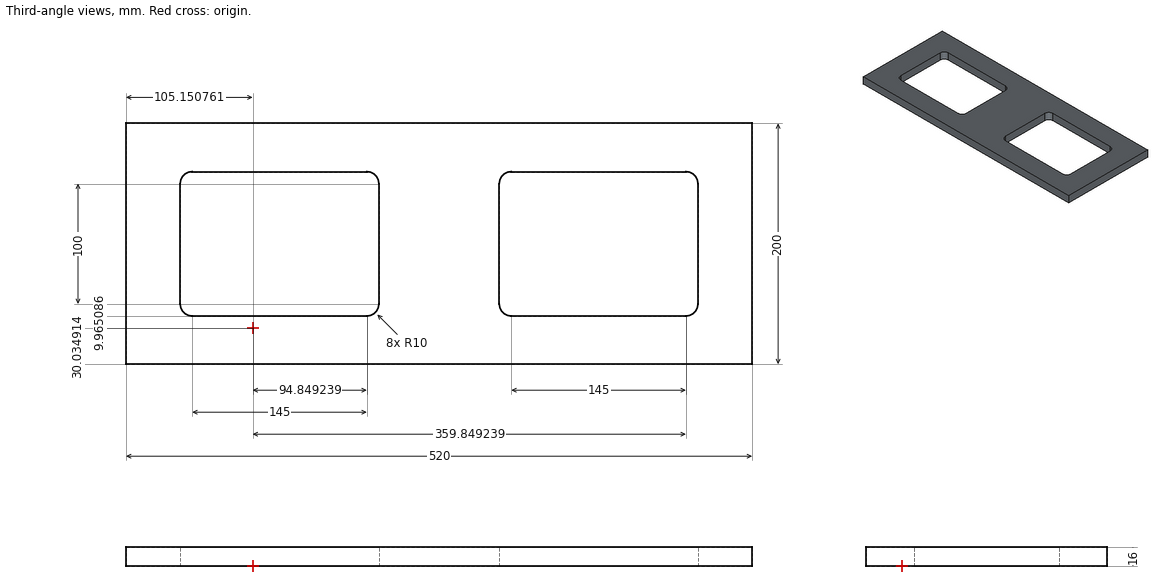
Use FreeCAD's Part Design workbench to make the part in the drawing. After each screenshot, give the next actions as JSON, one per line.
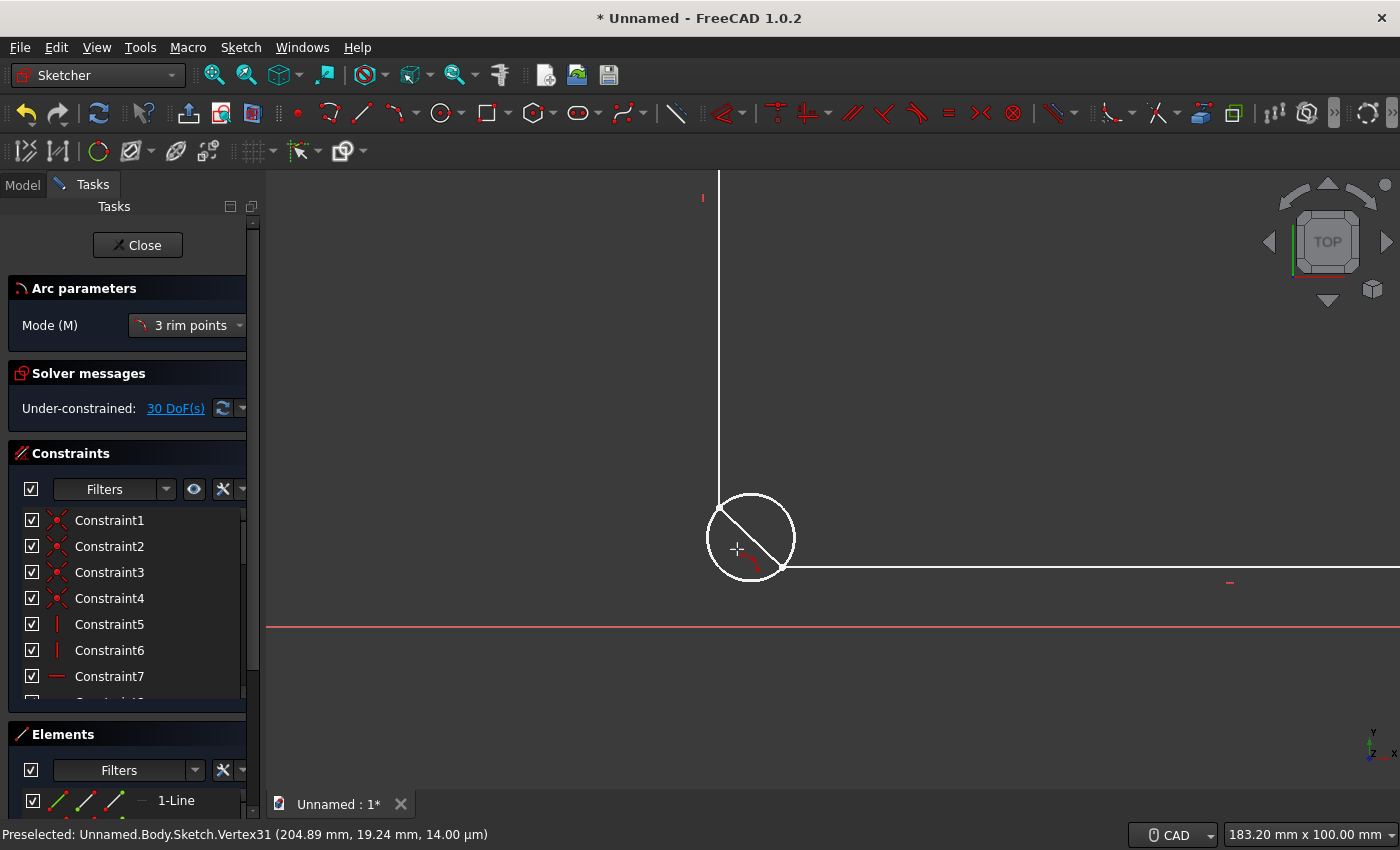
{"action": "left_click", "coordinate": [737, 547]}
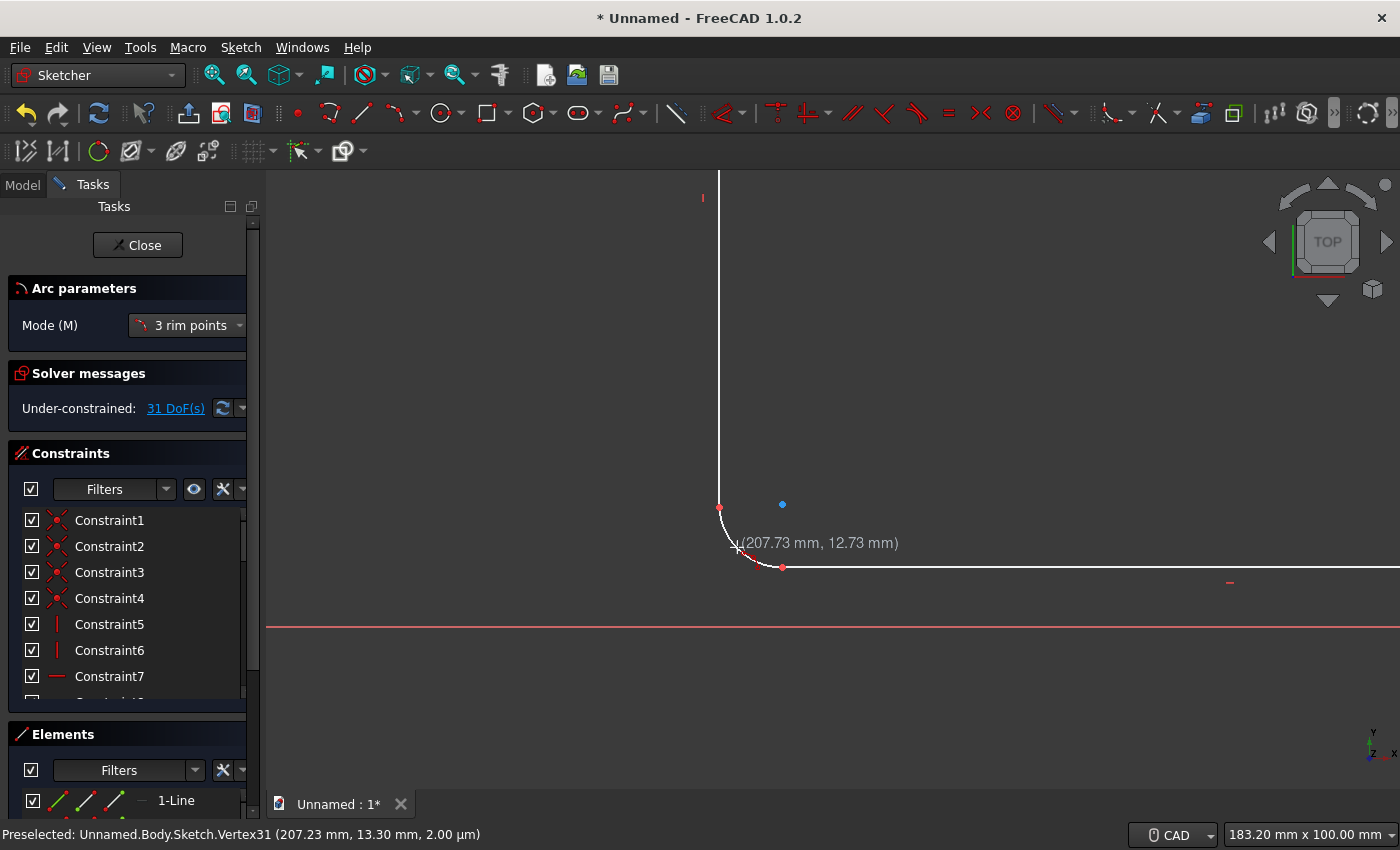
{"action": "scroll", "coordinate": [854, 552], "scroll_direction": "down", "scroll_amount": 8}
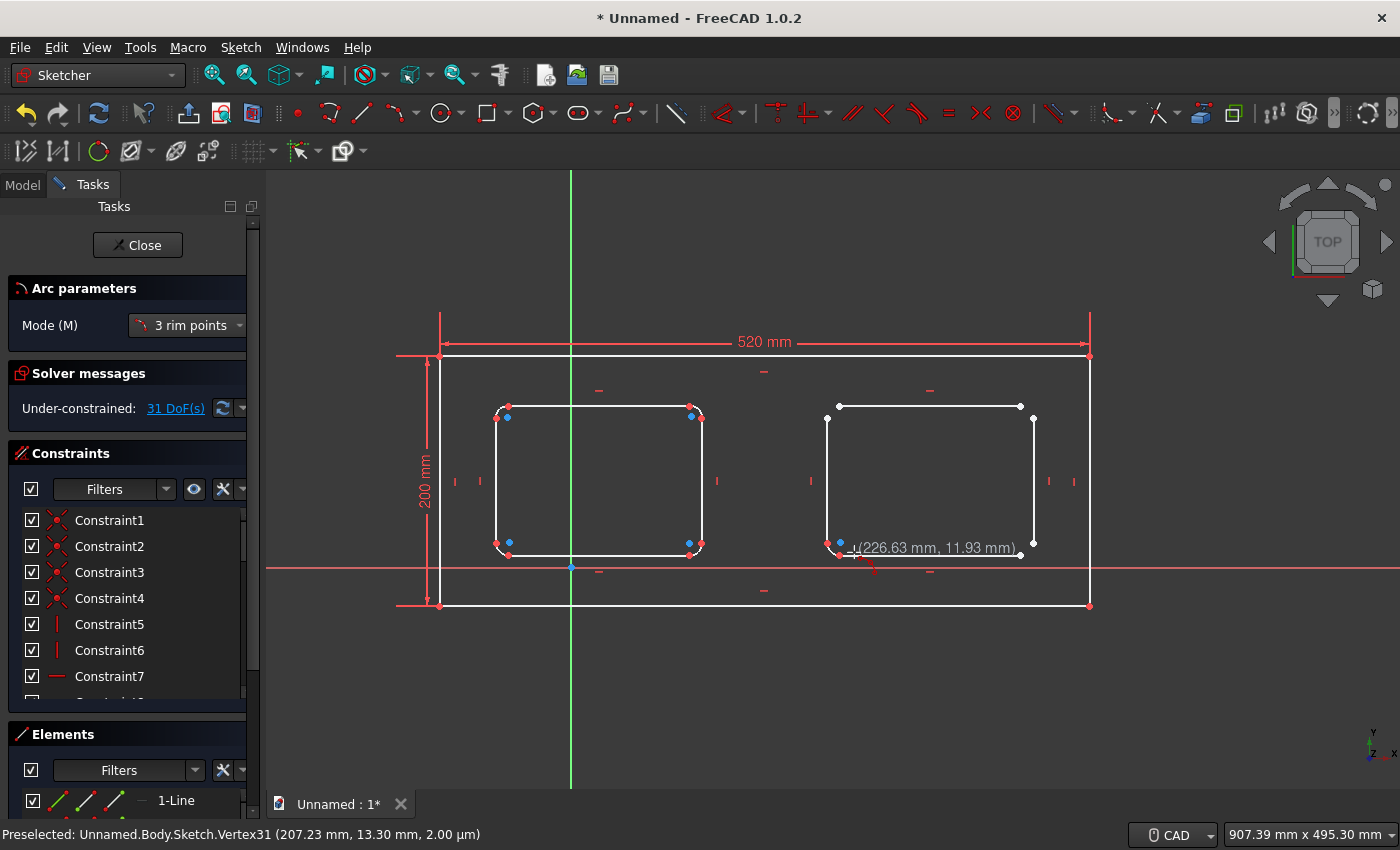
{"action": "left_click", "coordinate": [827, 418]}
{"action": "left_click", "coordinate": [840, 406]}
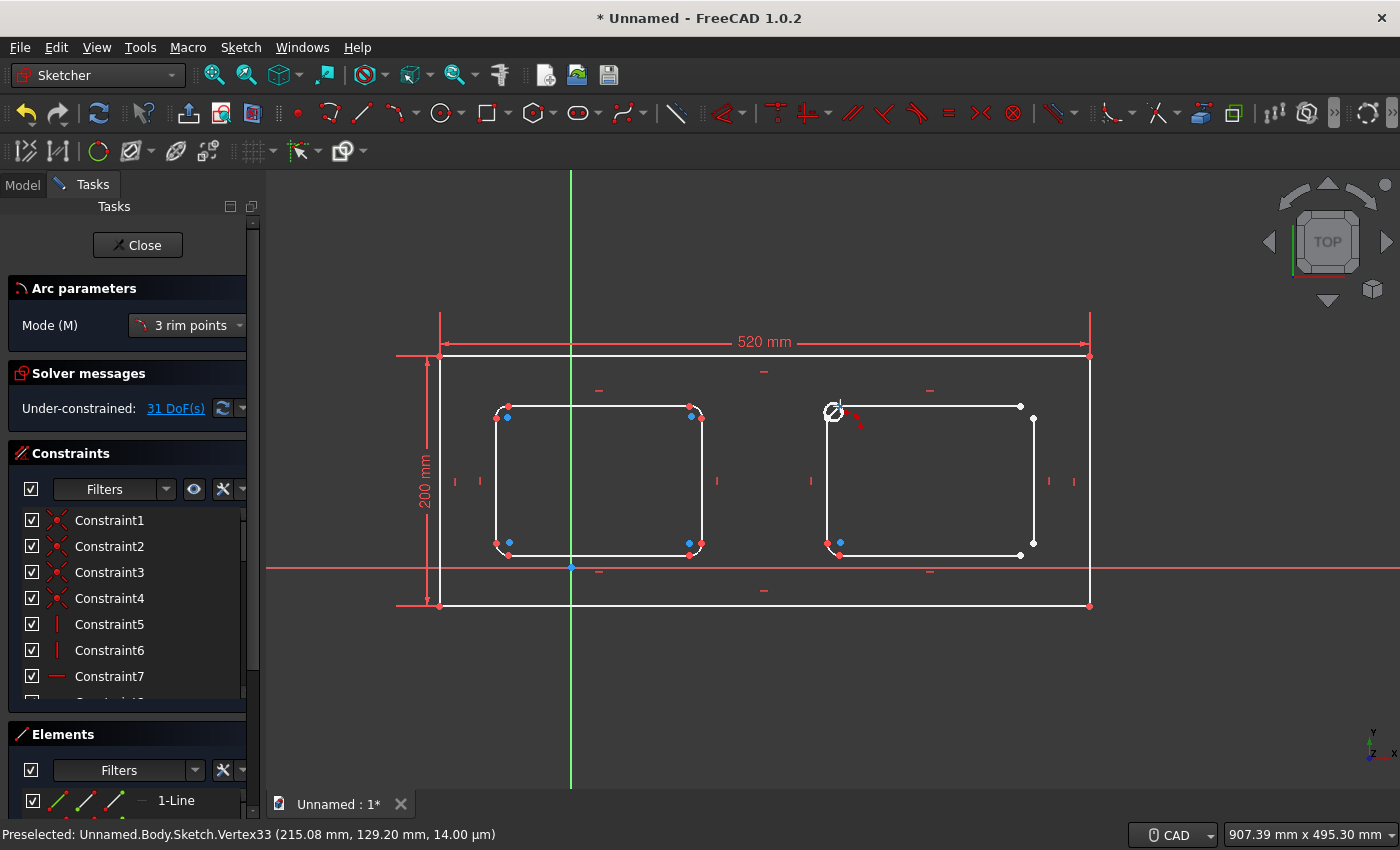
{"action": "scroll", "coordinate": [831, 409], "scroll_direction": "up", "scroll_amount": 8}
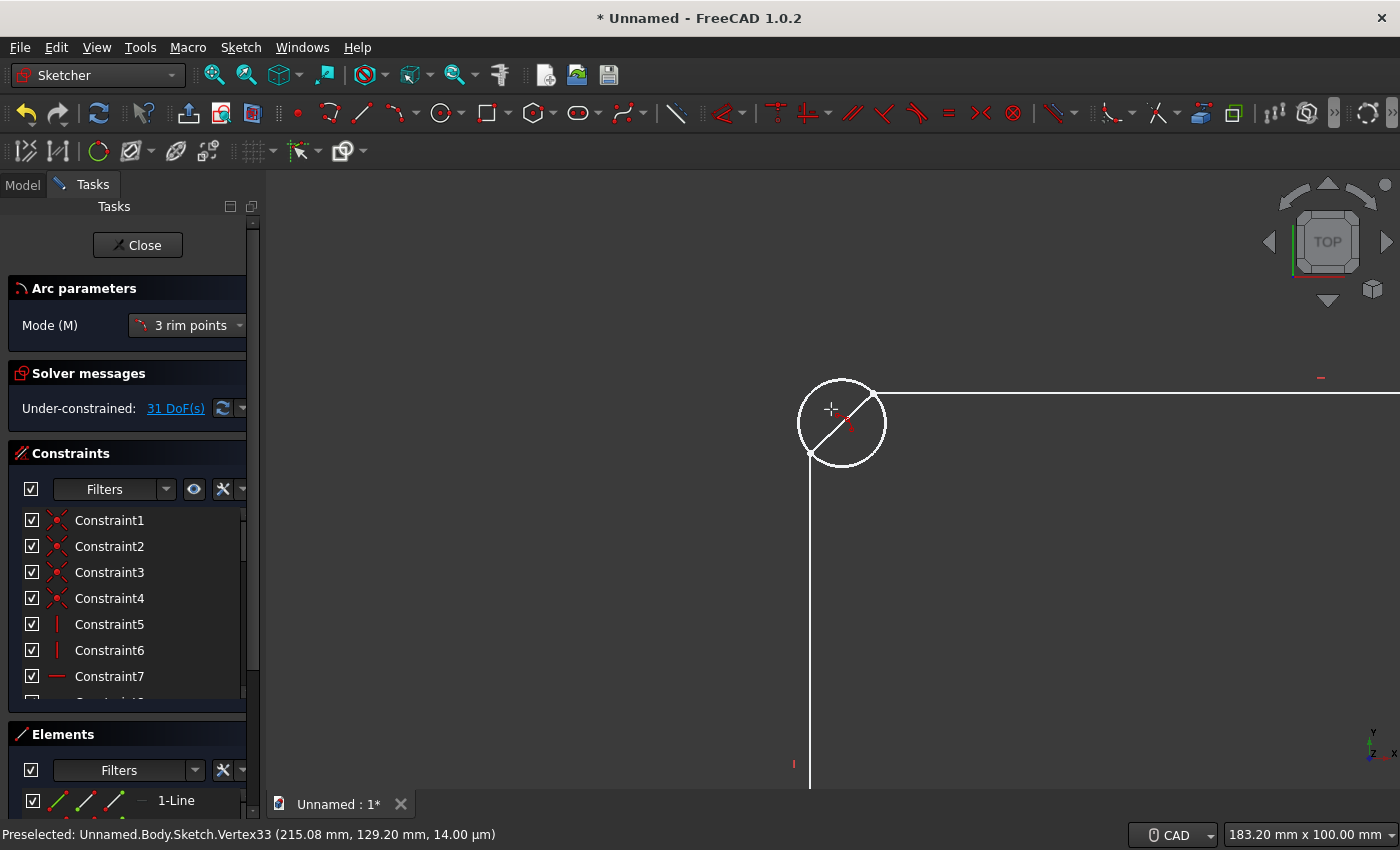
{"action": "left_click", "coordinate": [828, 407]}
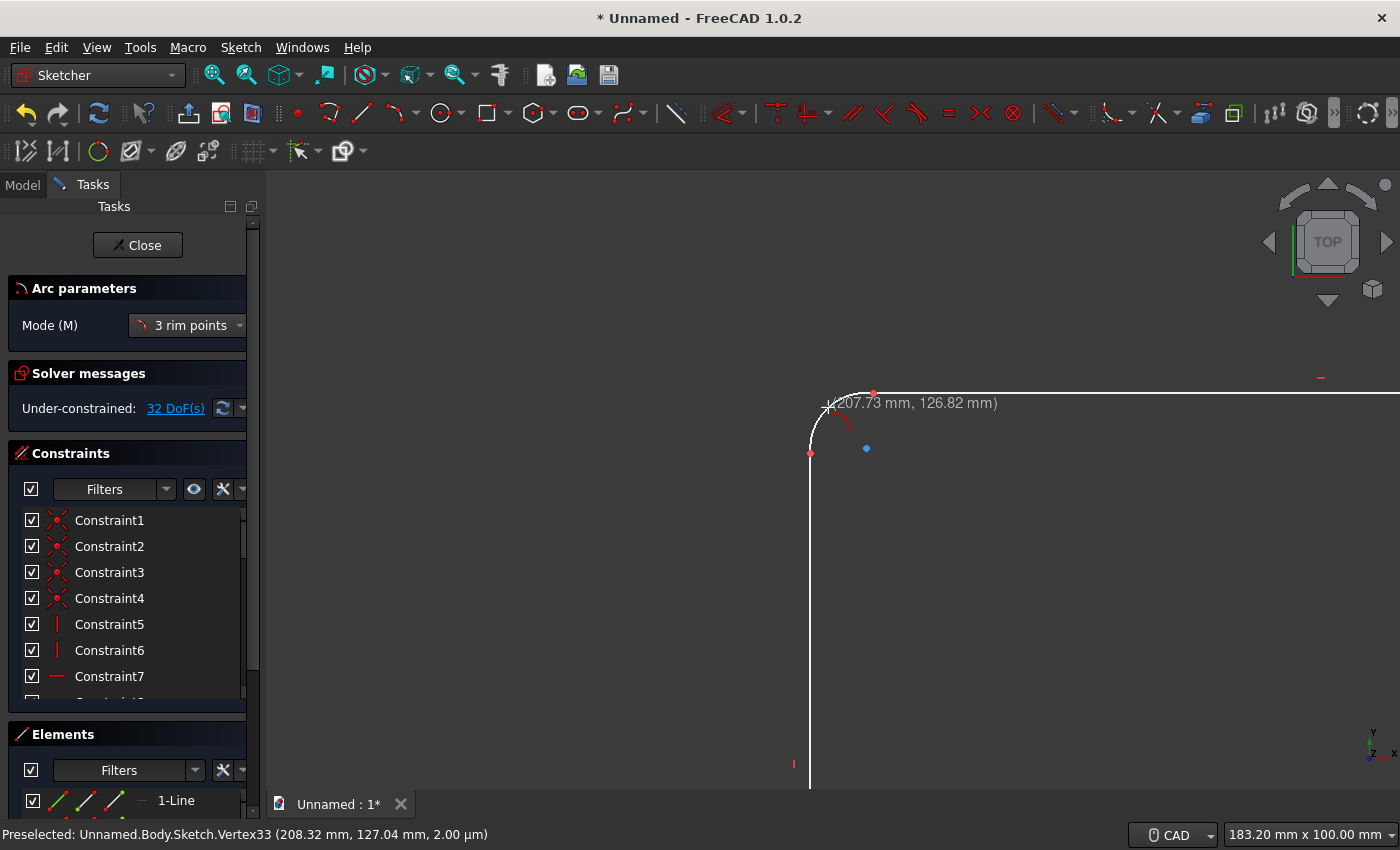
{"action": "scroll", "coordinate": [831, 409], "scroll_direction": "down", "scroll_amount": 8}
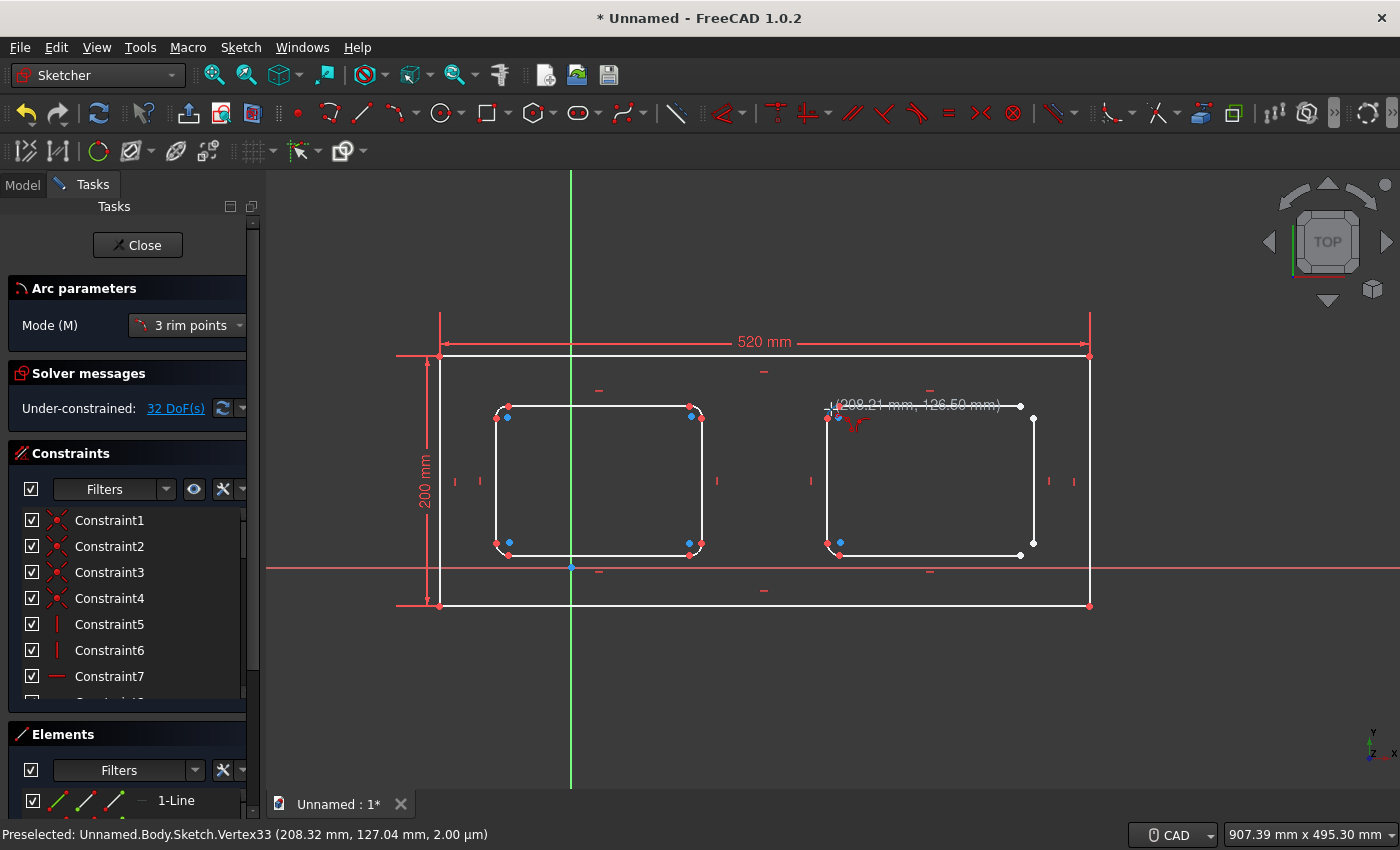
{"action": "left_click", "coordinate": [1021, 406]}
{"action": "left_click", "coordinate": [1034, 418]}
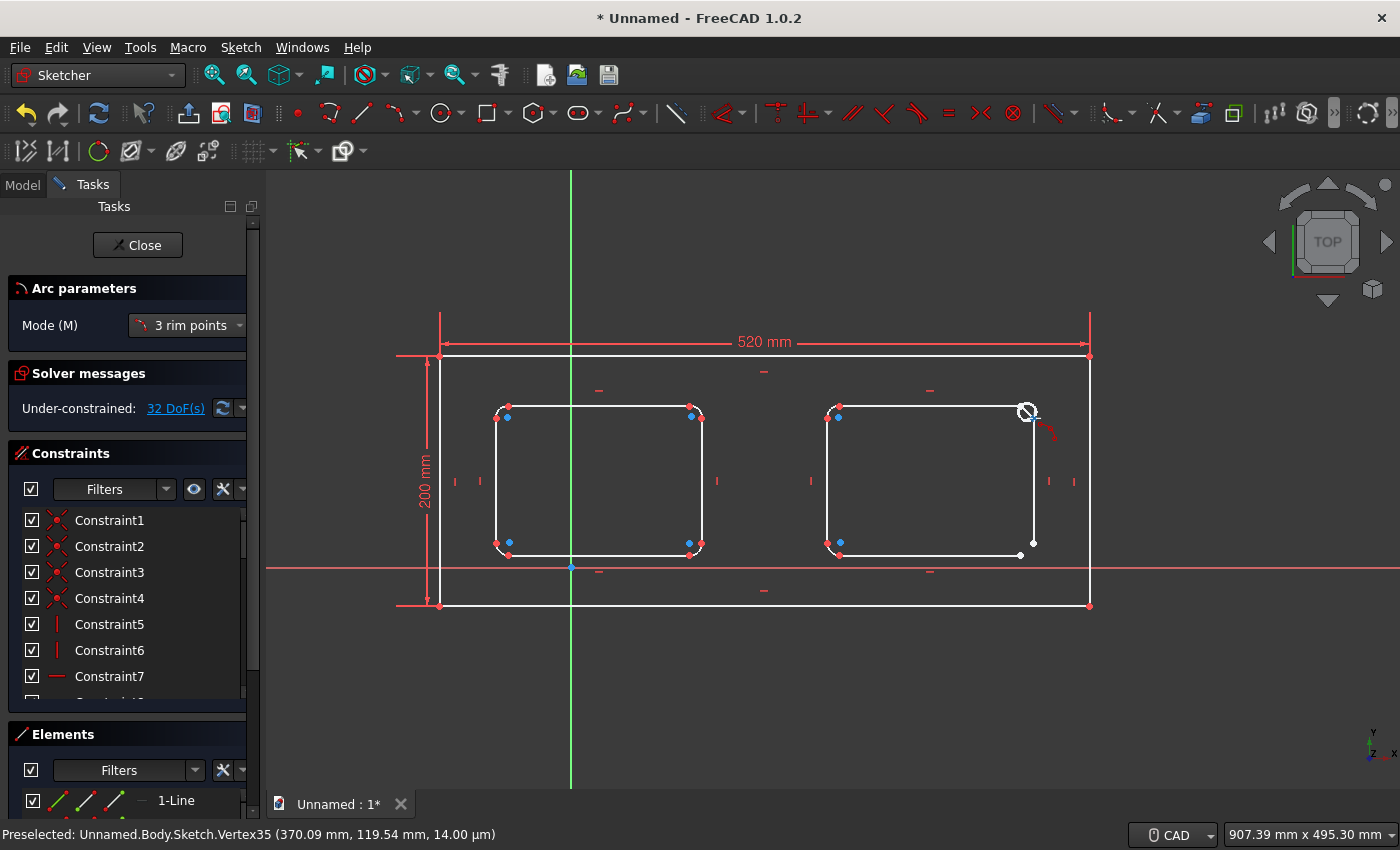
{"action": "scroll", "coordinate": [1030, 409], "scroll_direction": "up", "scroll_amount": 8}